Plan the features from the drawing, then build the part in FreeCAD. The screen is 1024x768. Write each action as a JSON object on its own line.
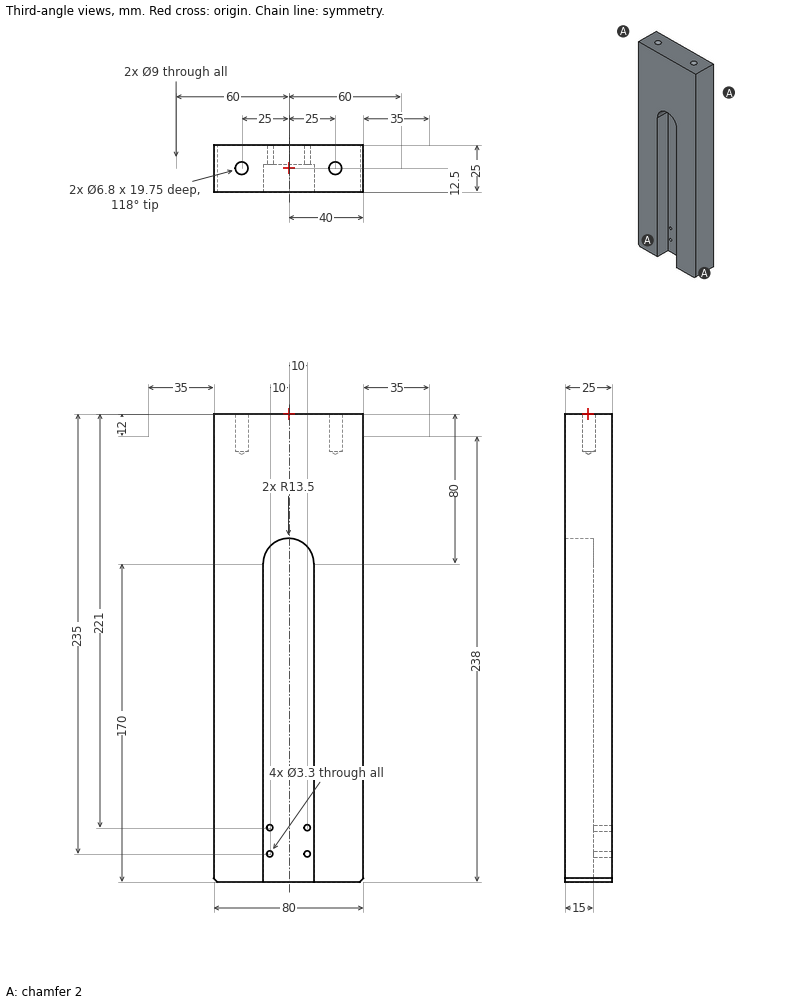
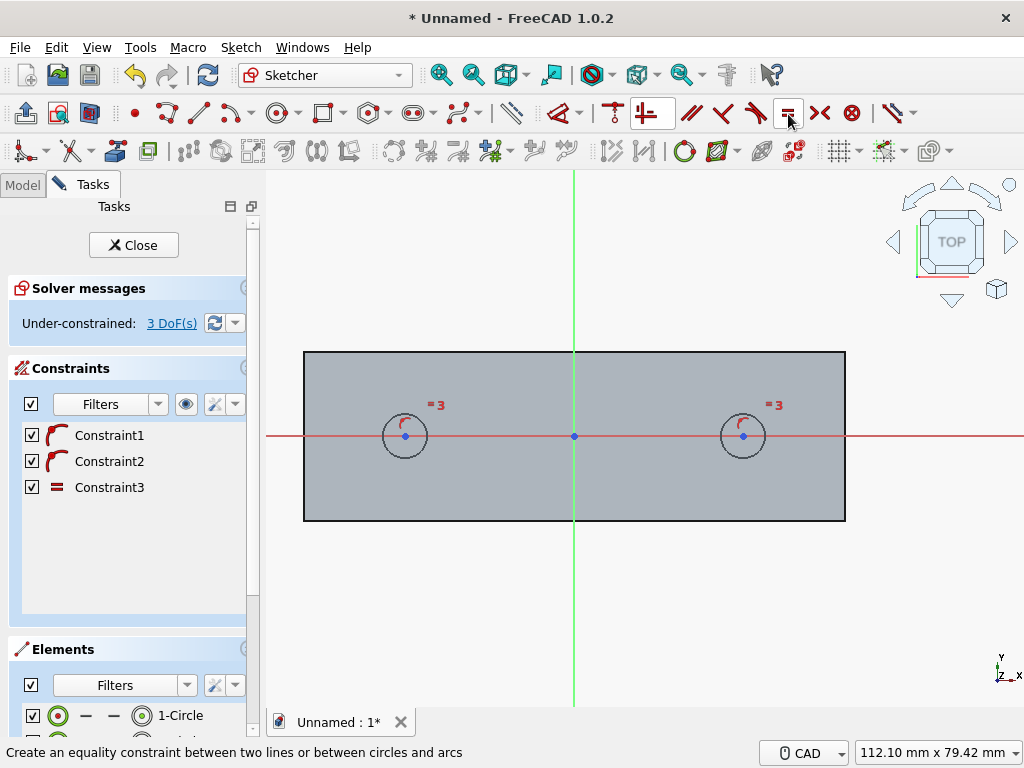
{"action": "left_click", "coordinate": [558, 114]}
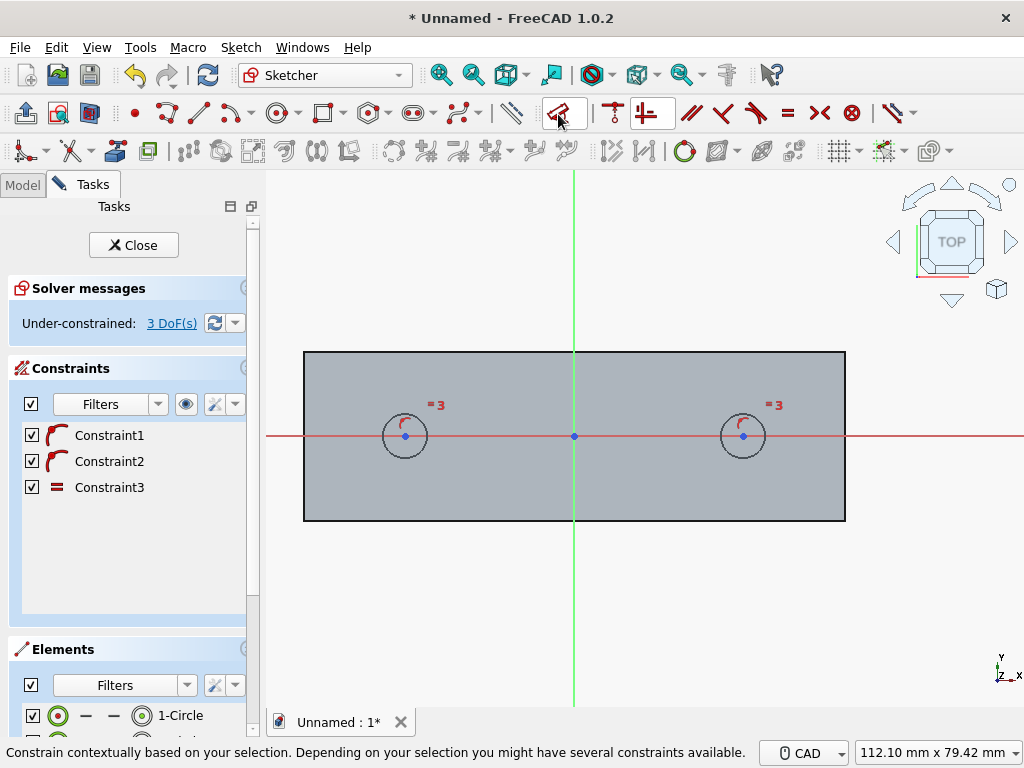
{"action": "left_click", "coordinate": [421, 421]}
{"action": "left_click", "coordinate": [444, 399]}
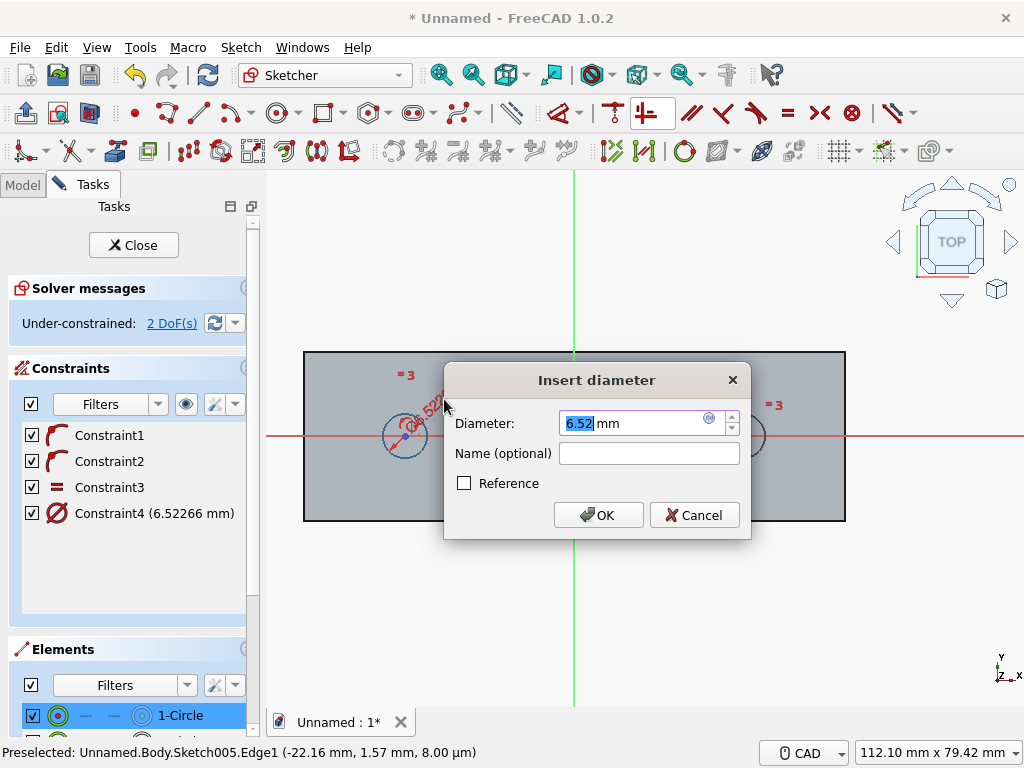
{"action": "type", "text": "6.8"}
{"action": "key", "text": "Return"}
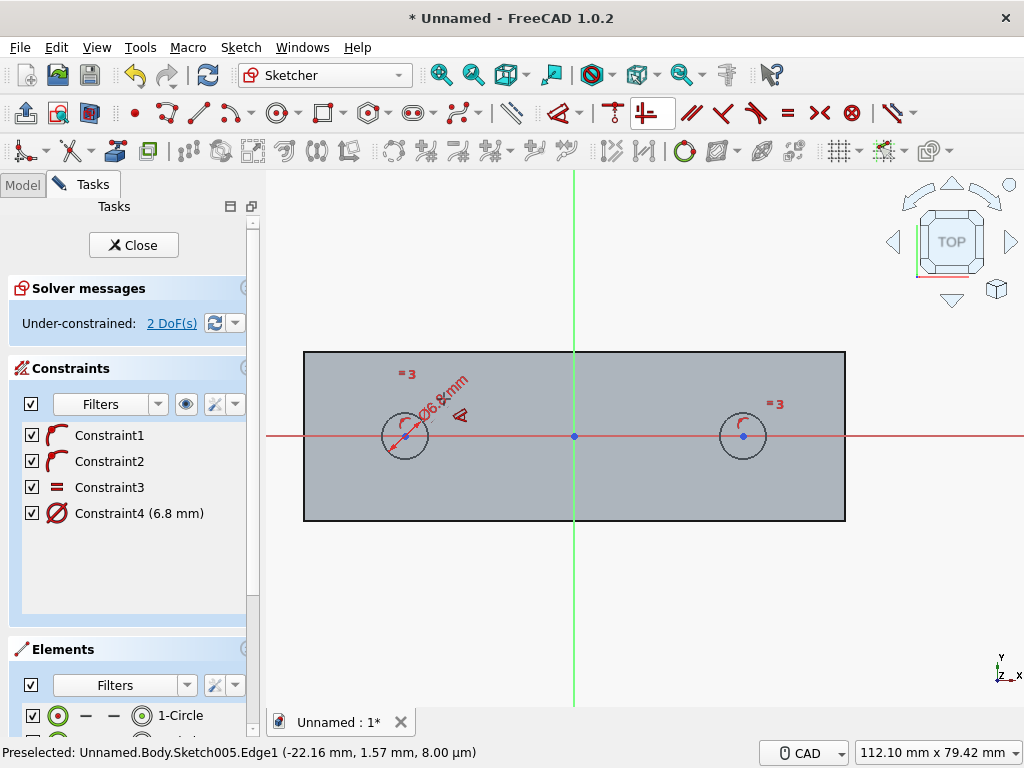
{"action": "left_click", "coordinate": [405, 436]}
{"action": "left_click", "coordinate": [490, 470]}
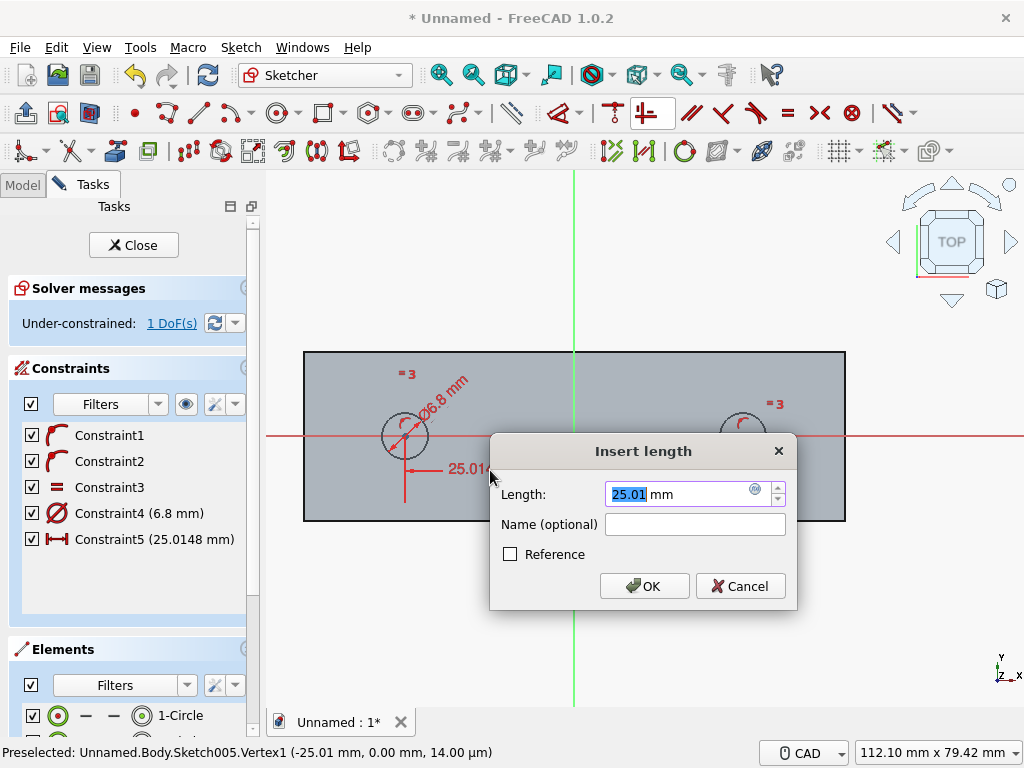
{"action": "type", "text": "25"}
{"action": "key", "text": "Return"}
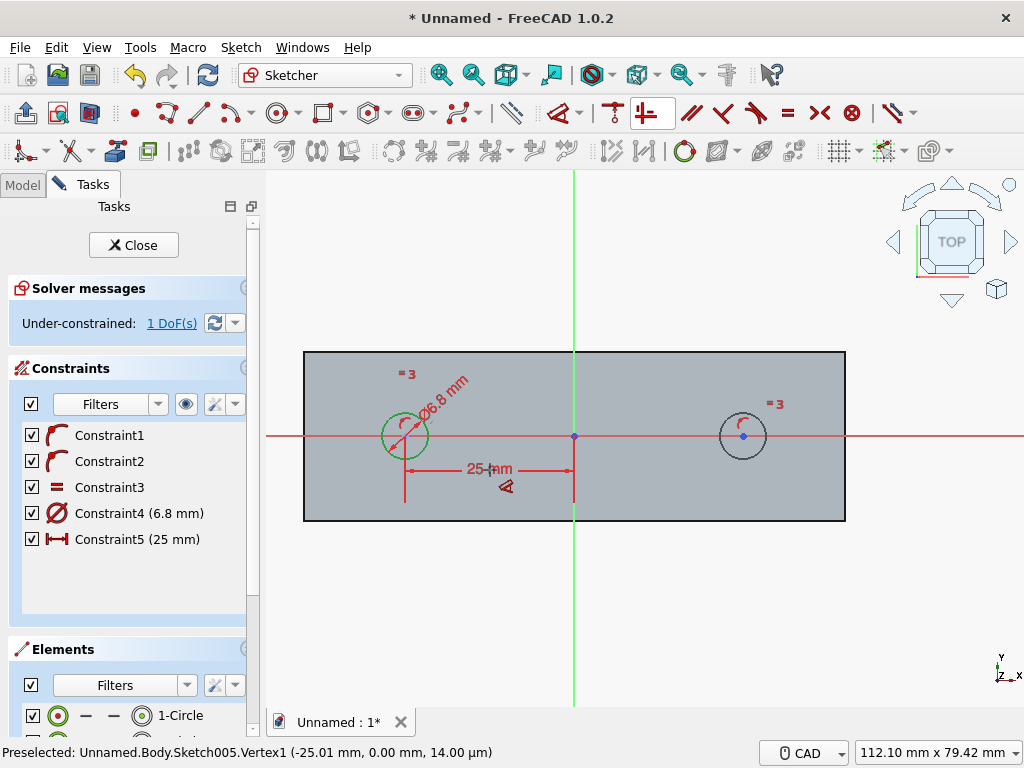
{"action": "left_click", "coordinate": [743, 436]}
{"action": "left_click", "coordinate": [659, 470]}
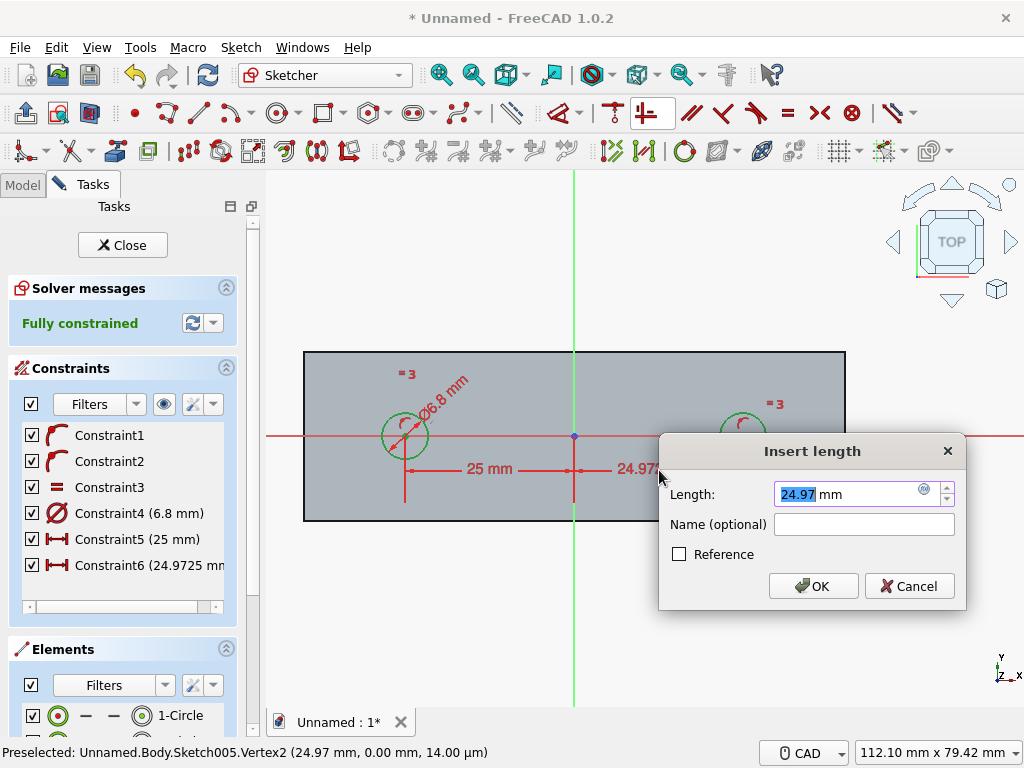
{"action": "type", "text": "25"}
{"action": "key", "text": "Return"}
{"action": "key", "text": "Escape"}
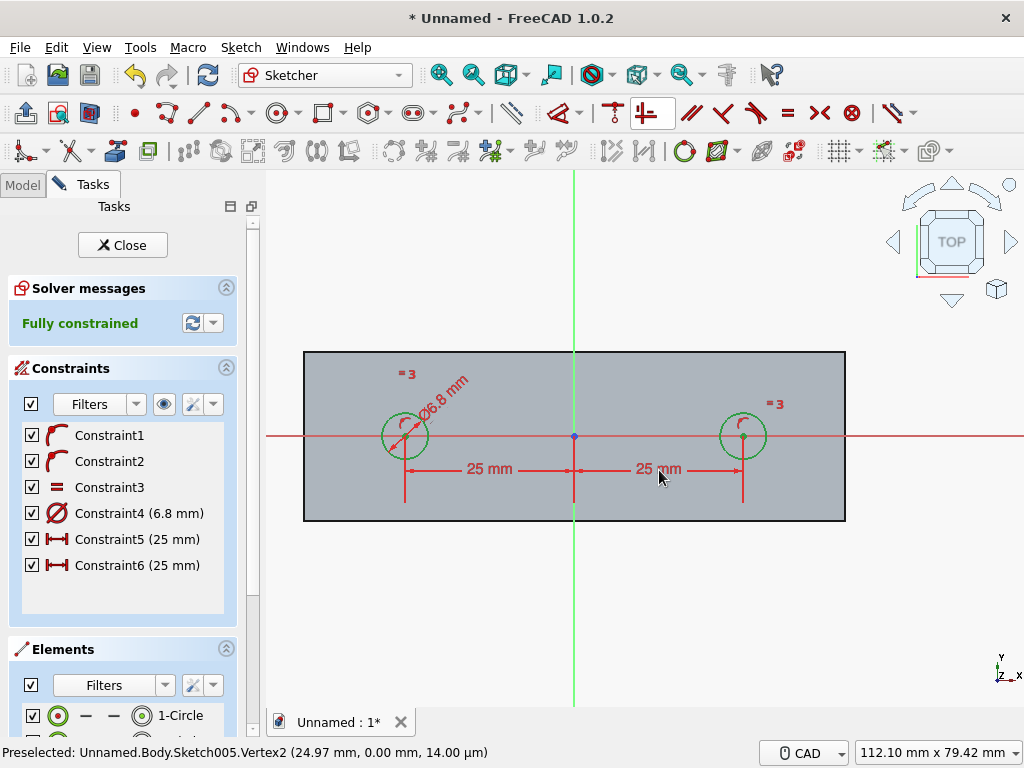
{"action": "left_click", "coordinate": [123, 245]}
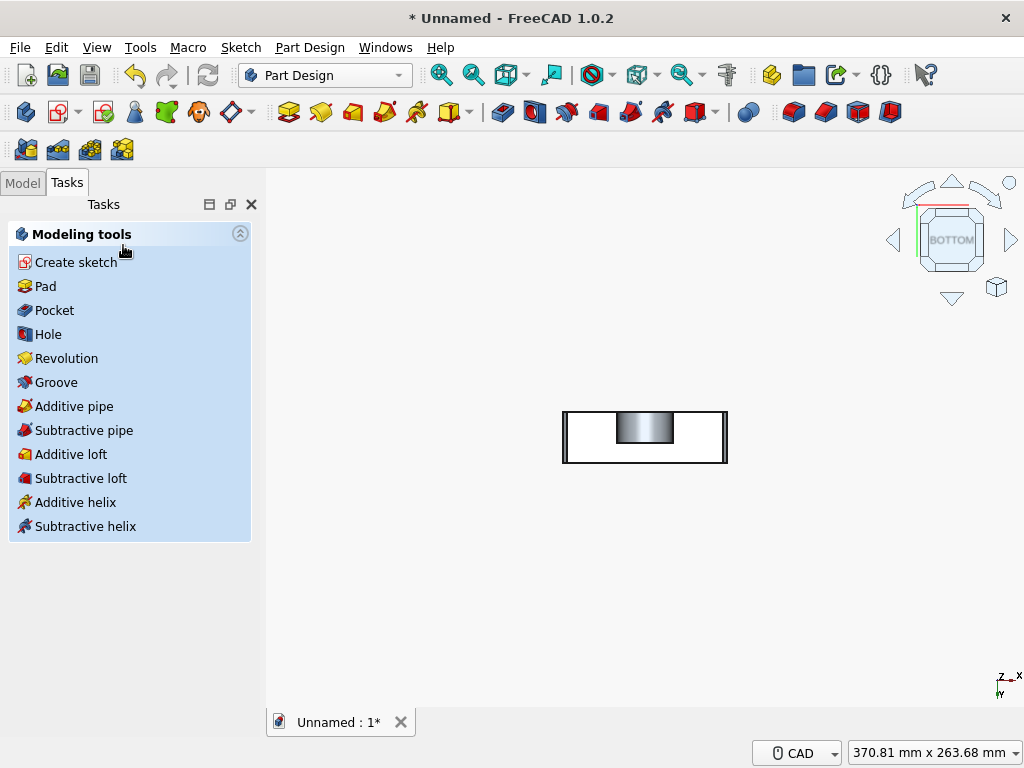
{"action": "left_click", "coordinate": [536, 112]}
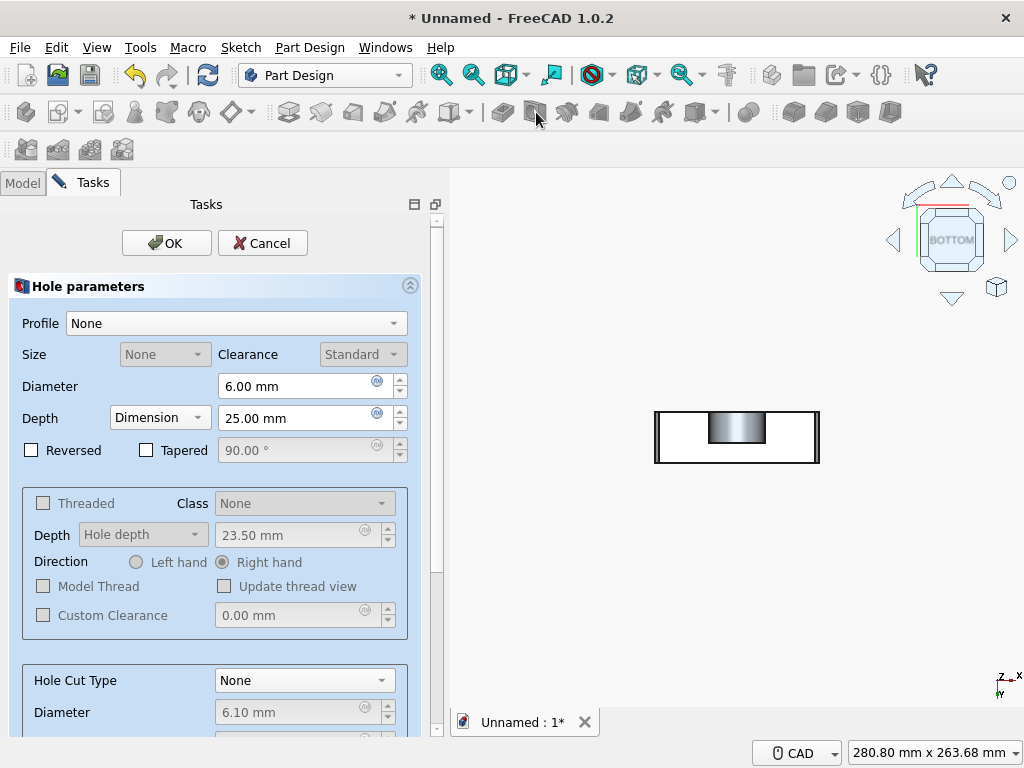
{"action": "triple_click", "coordinate": [305, 386]}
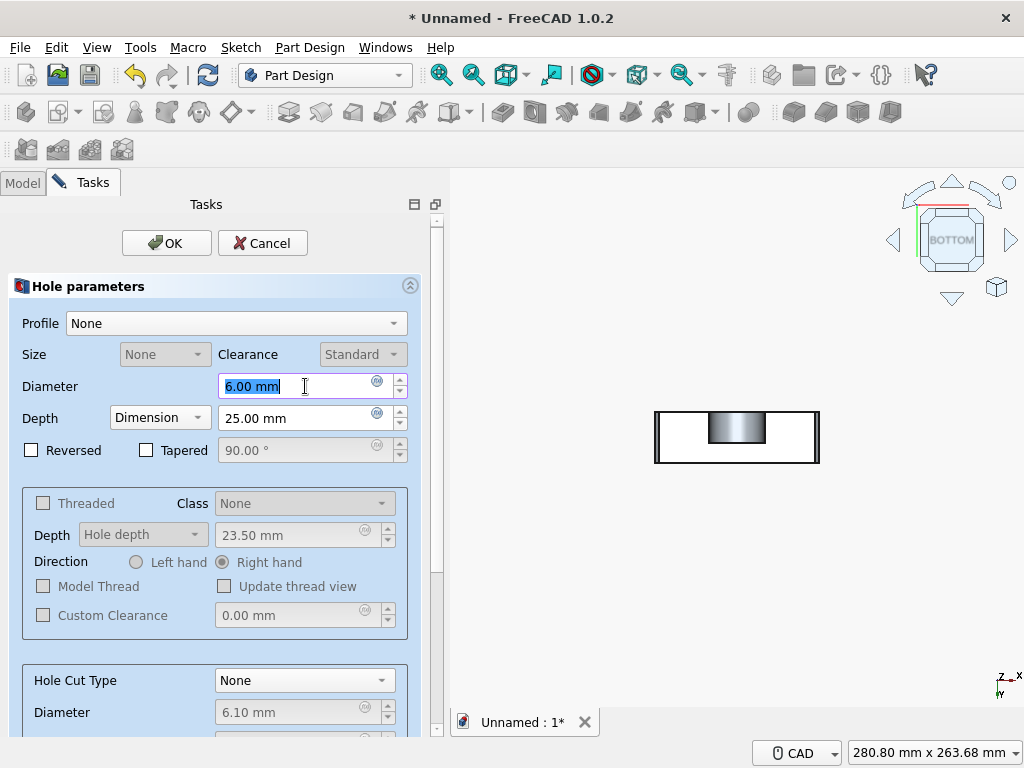
{"action": "type", "text": "6.8"}
{"action": "key", "text": "Tab"}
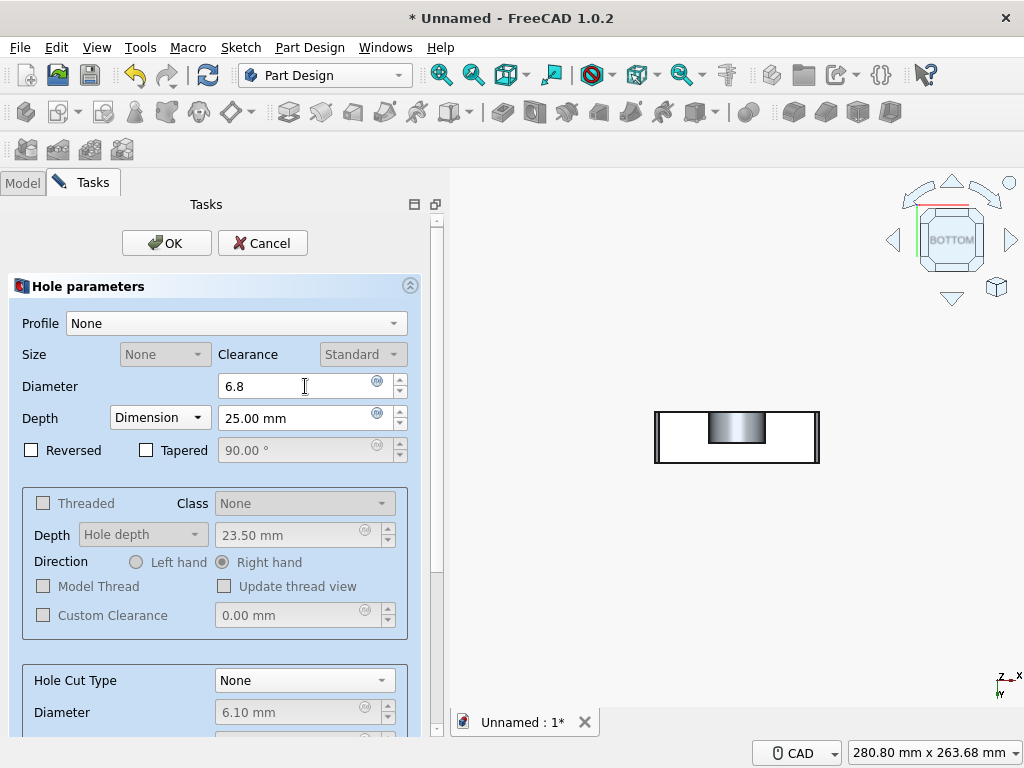
{"action": "triple_click", "coordinate": [305, 418]}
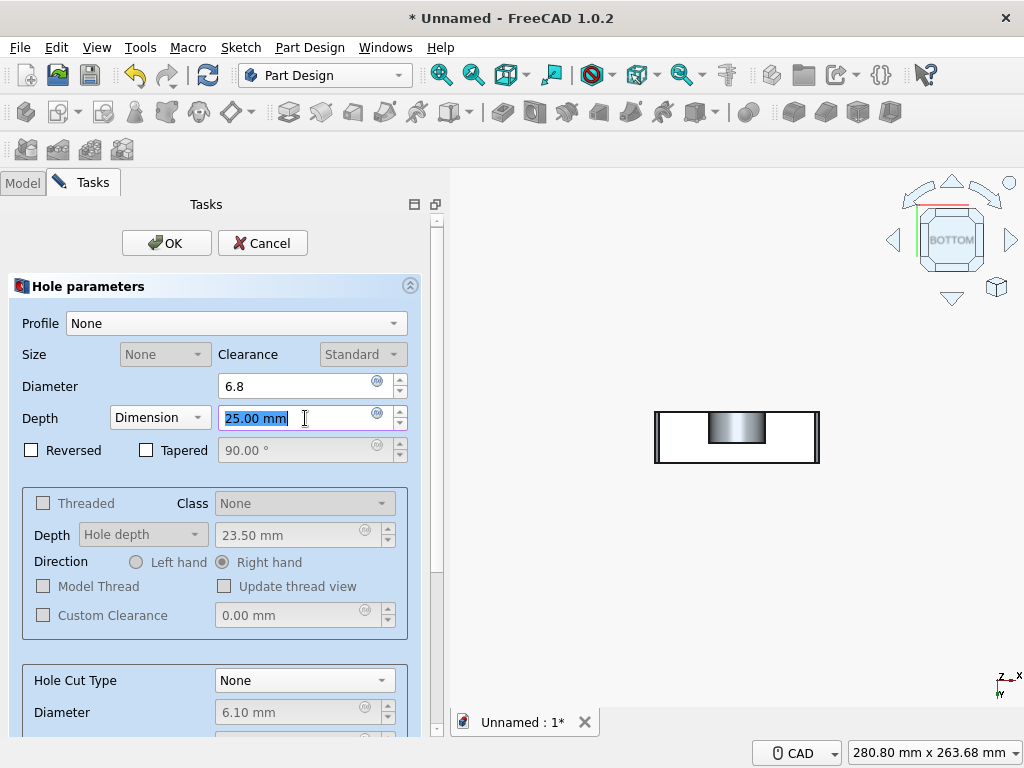
{"action": "type", "text": "19.75"}
{"action": "key", "text": "Tab"}